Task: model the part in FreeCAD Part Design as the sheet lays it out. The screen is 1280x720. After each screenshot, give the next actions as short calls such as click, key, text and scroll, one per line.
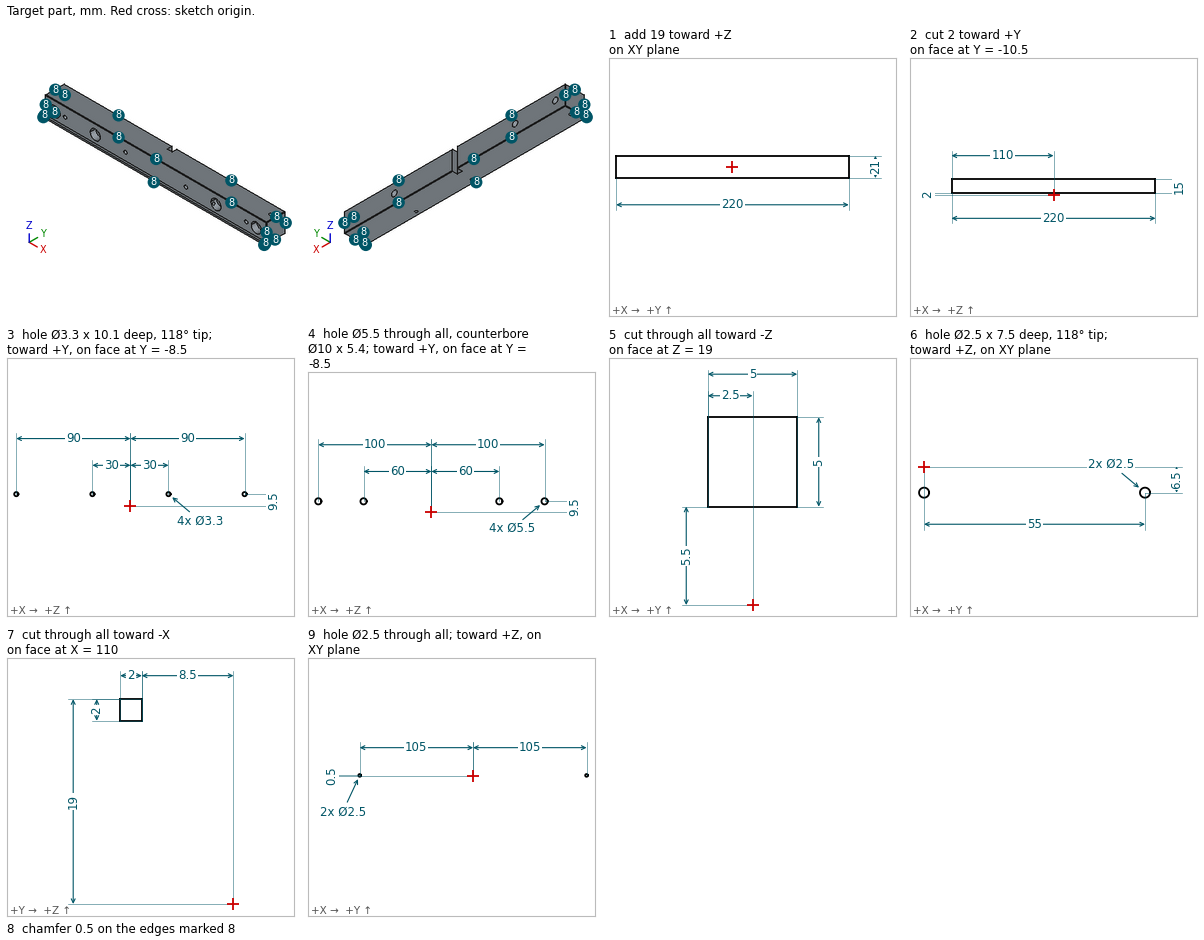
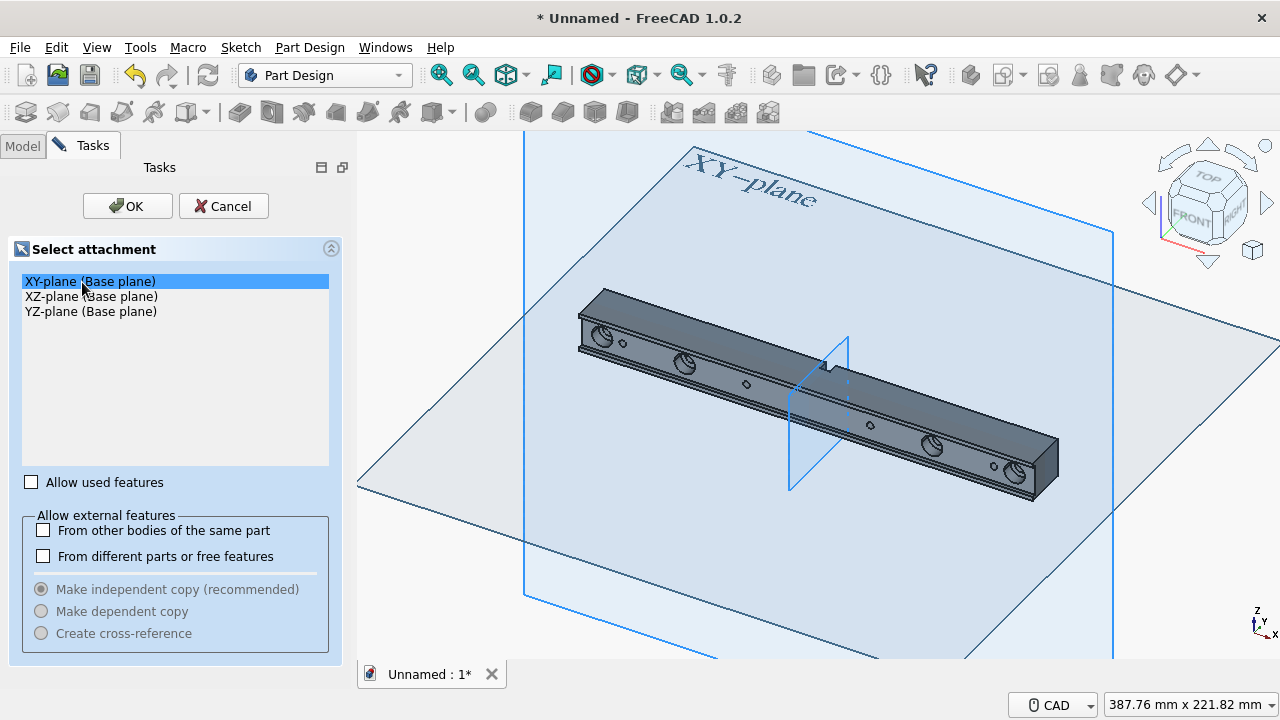
click(128, 206)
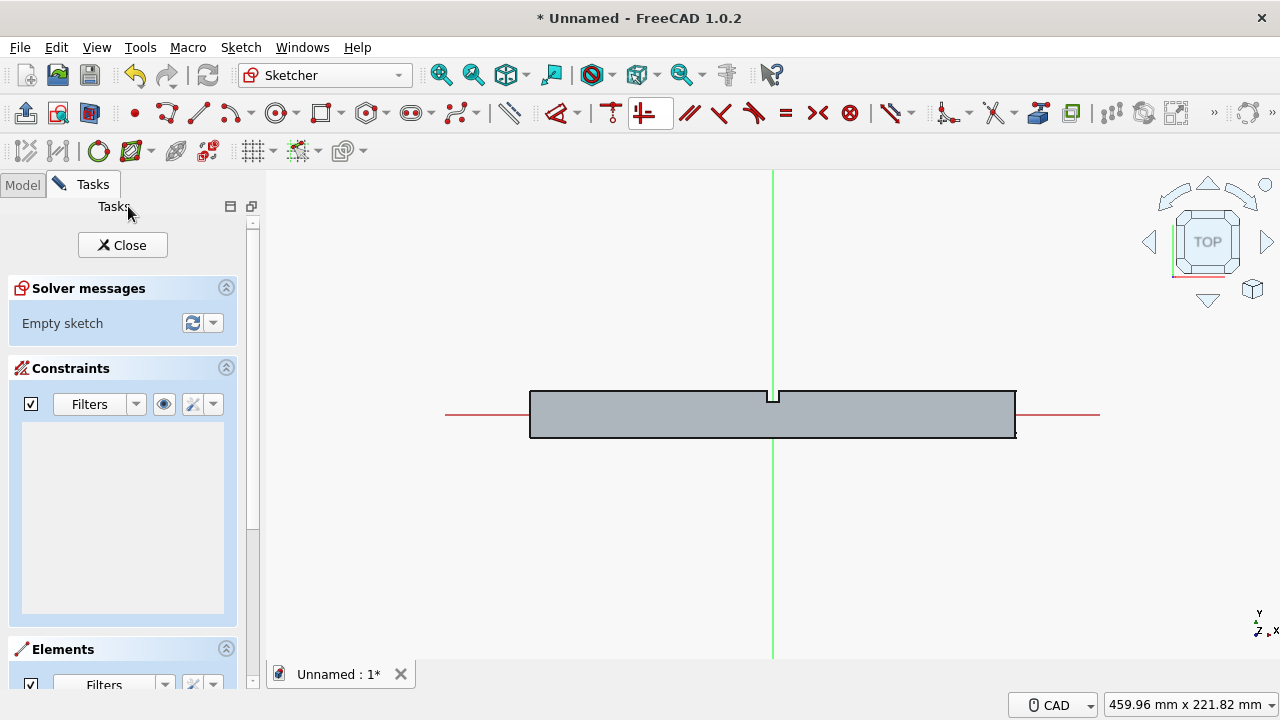
click(90, 114)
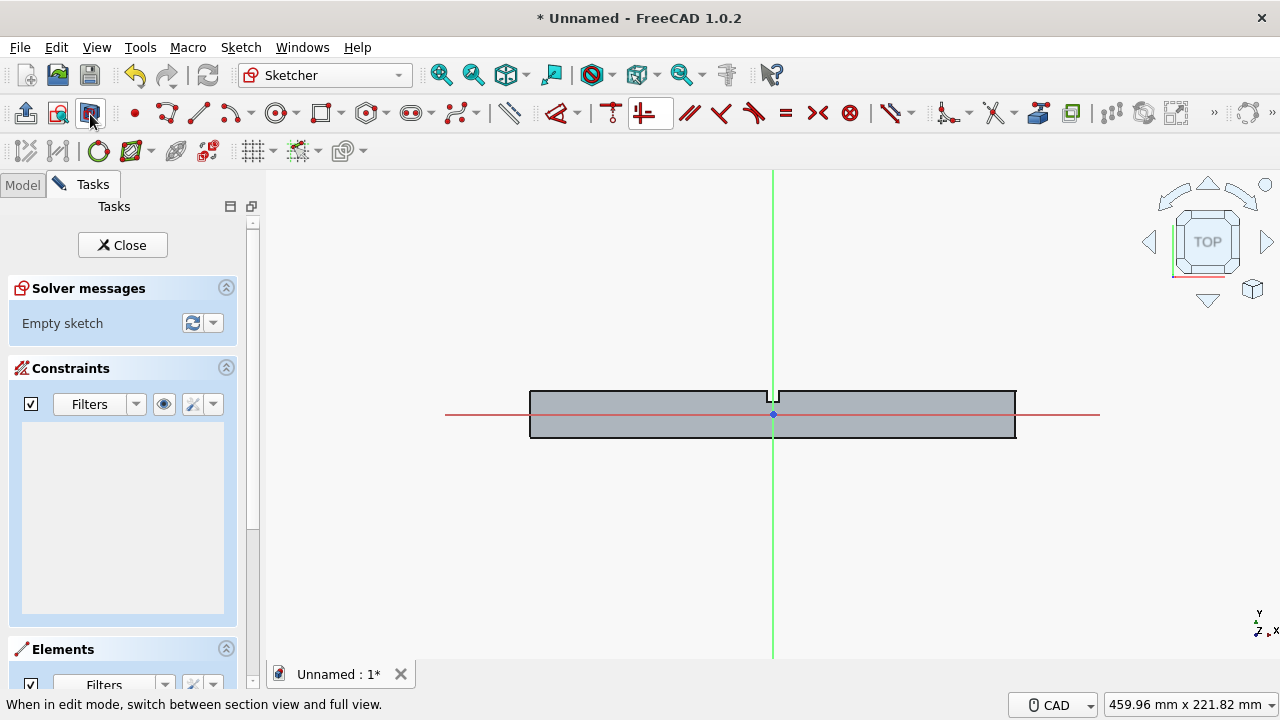
scroll(866, 425, up, 8)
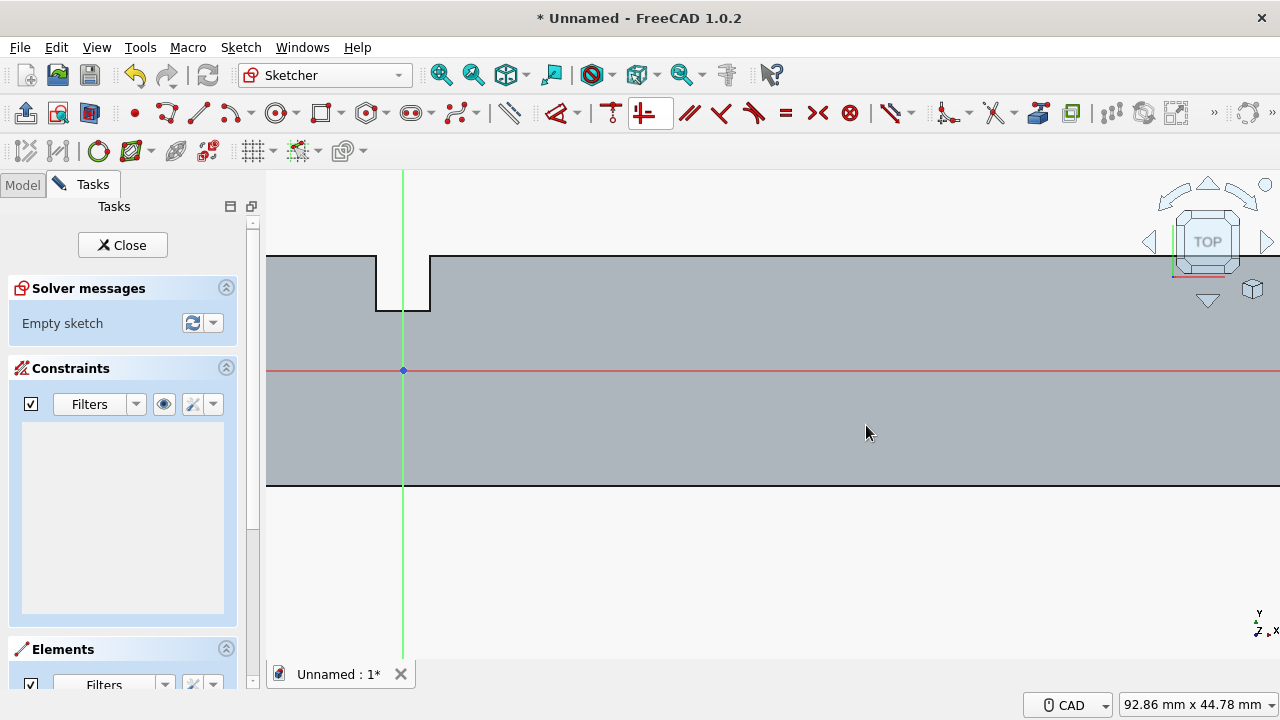
click(276, 114)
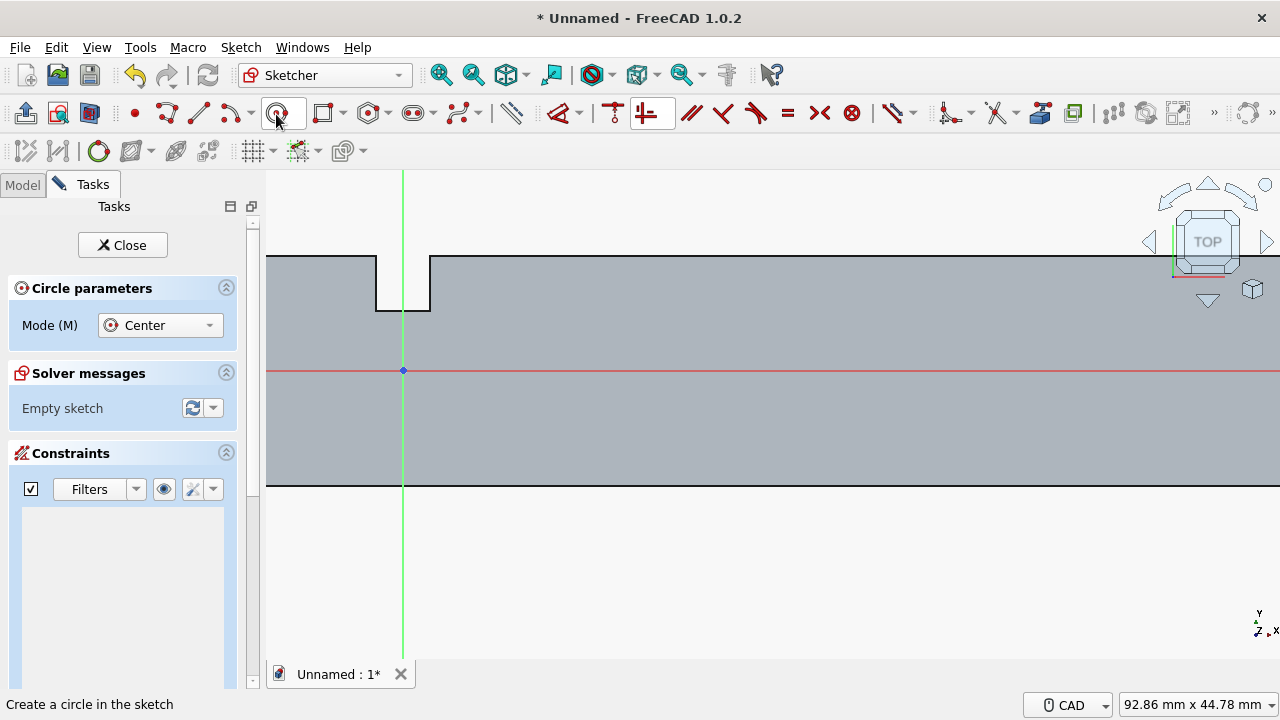
scroll(1004, 442, up, 3)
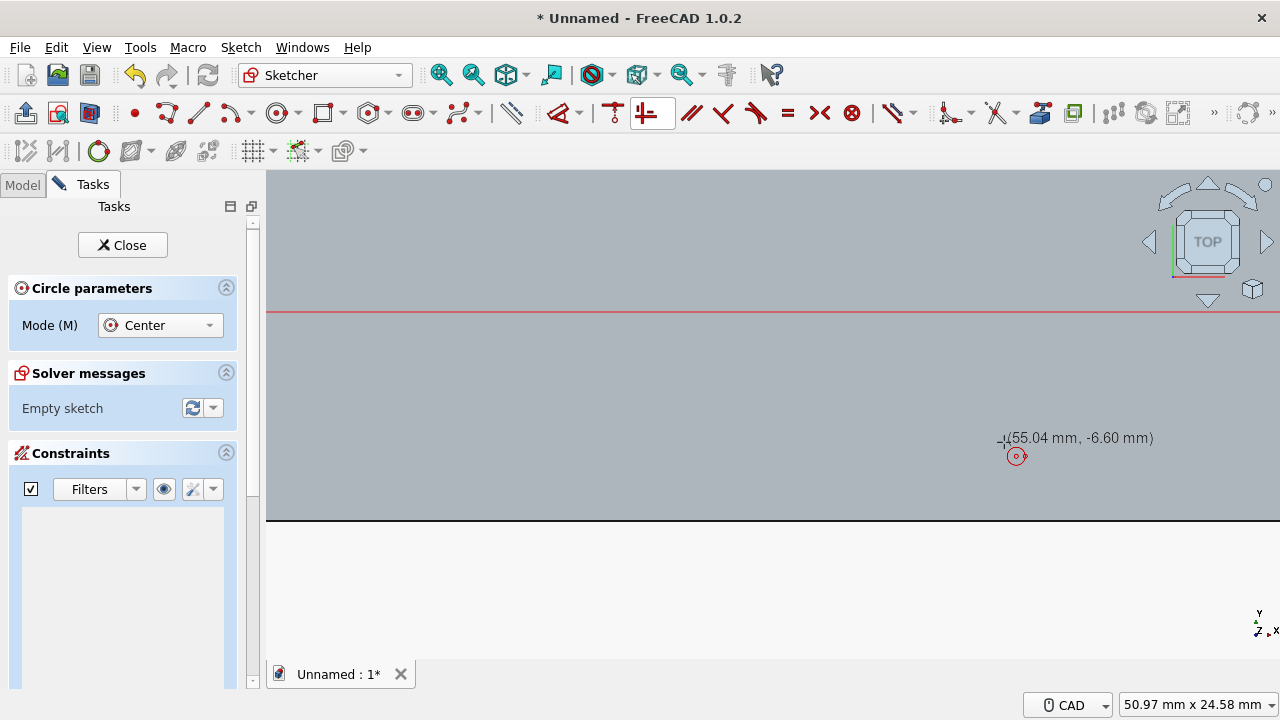
click(1003, 441)
move(1020, 424)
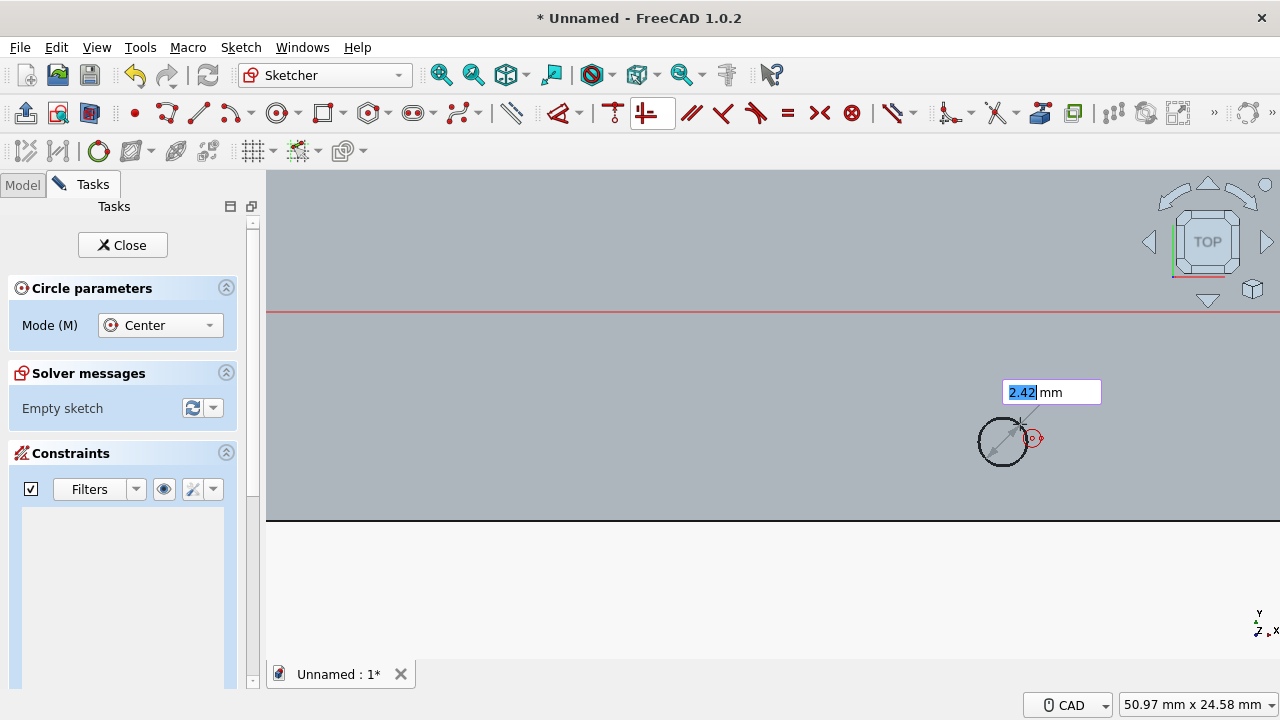
text(2.5)
key(Return)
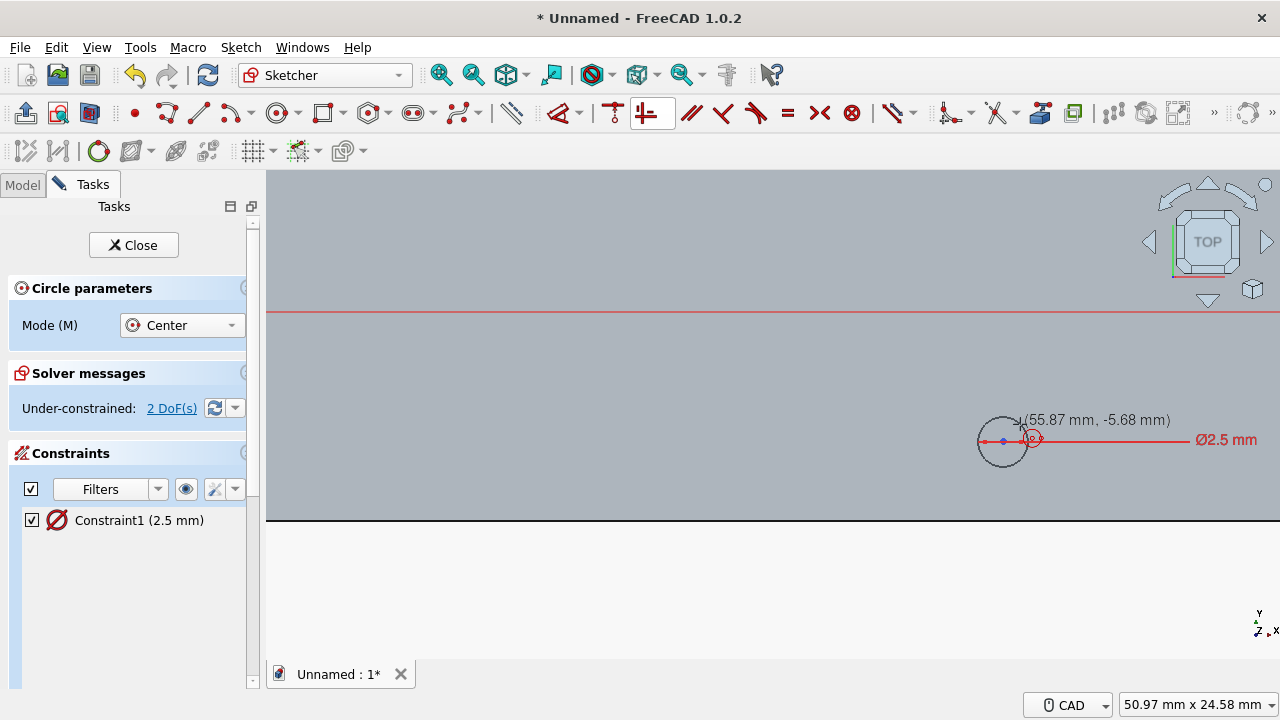
scroll(1007, 445, down, 3)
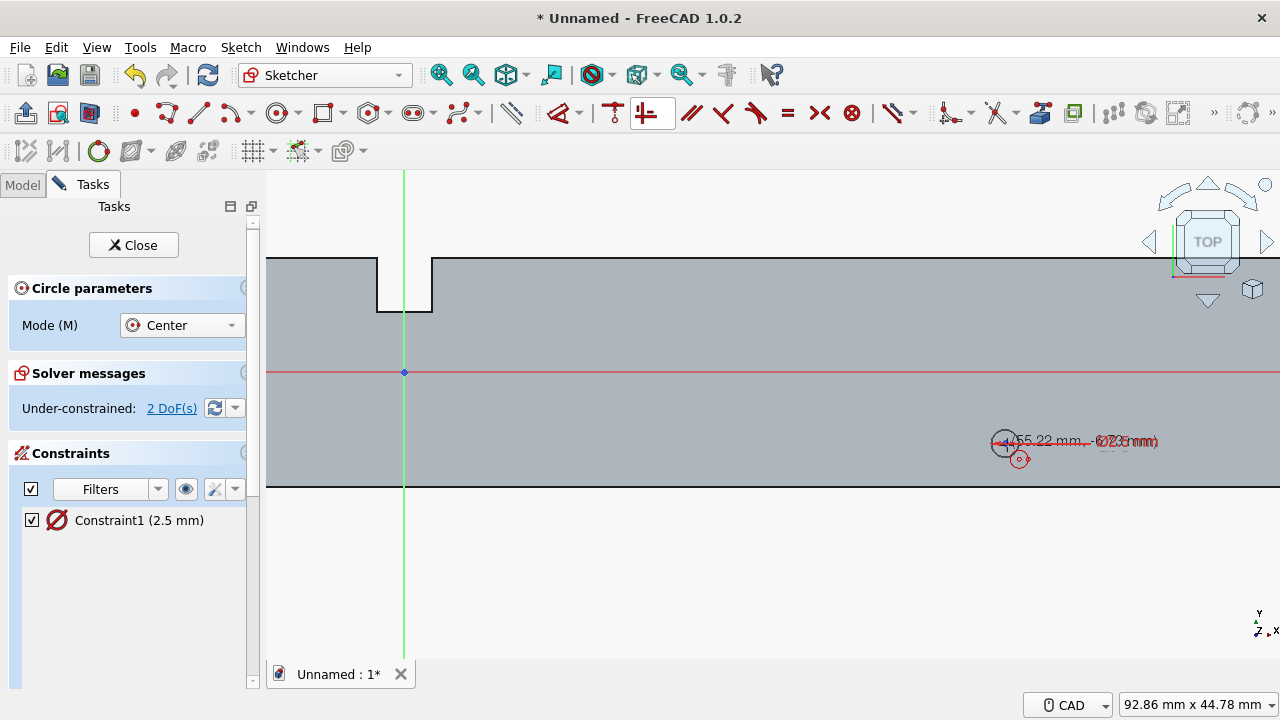
scroll(404, 443, up, 3)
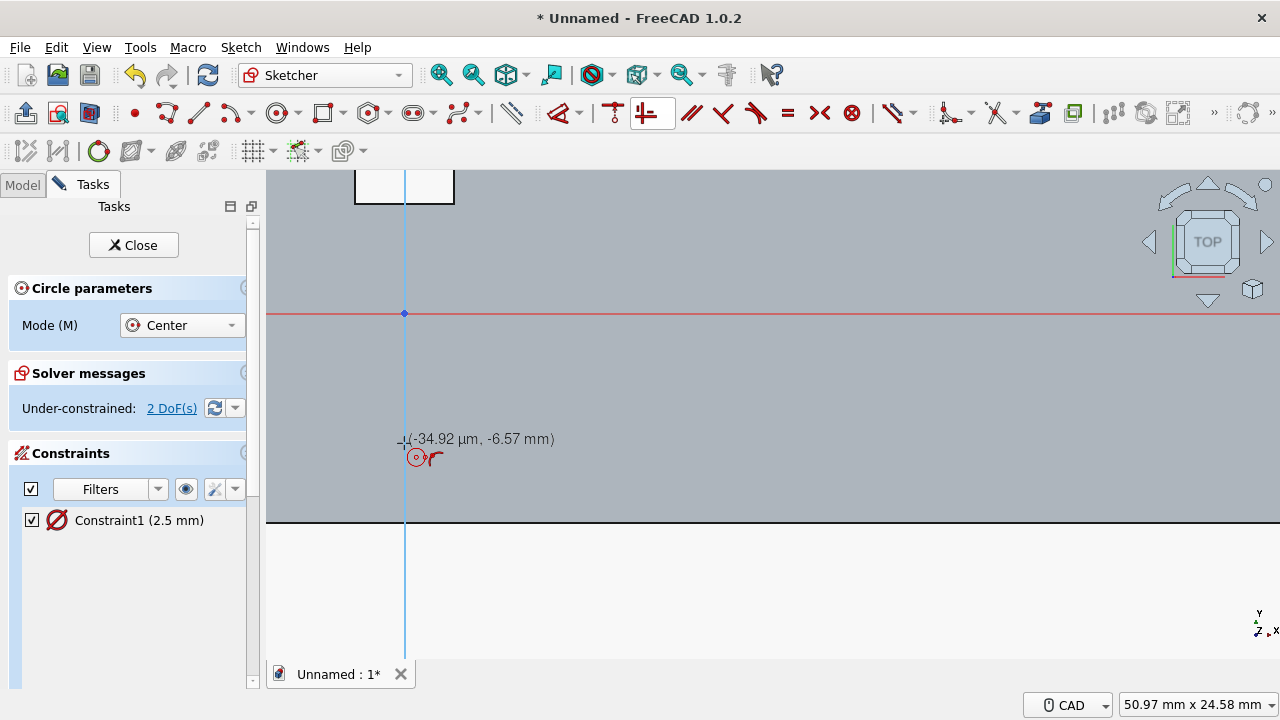
click(405, 443)
move(422, 425)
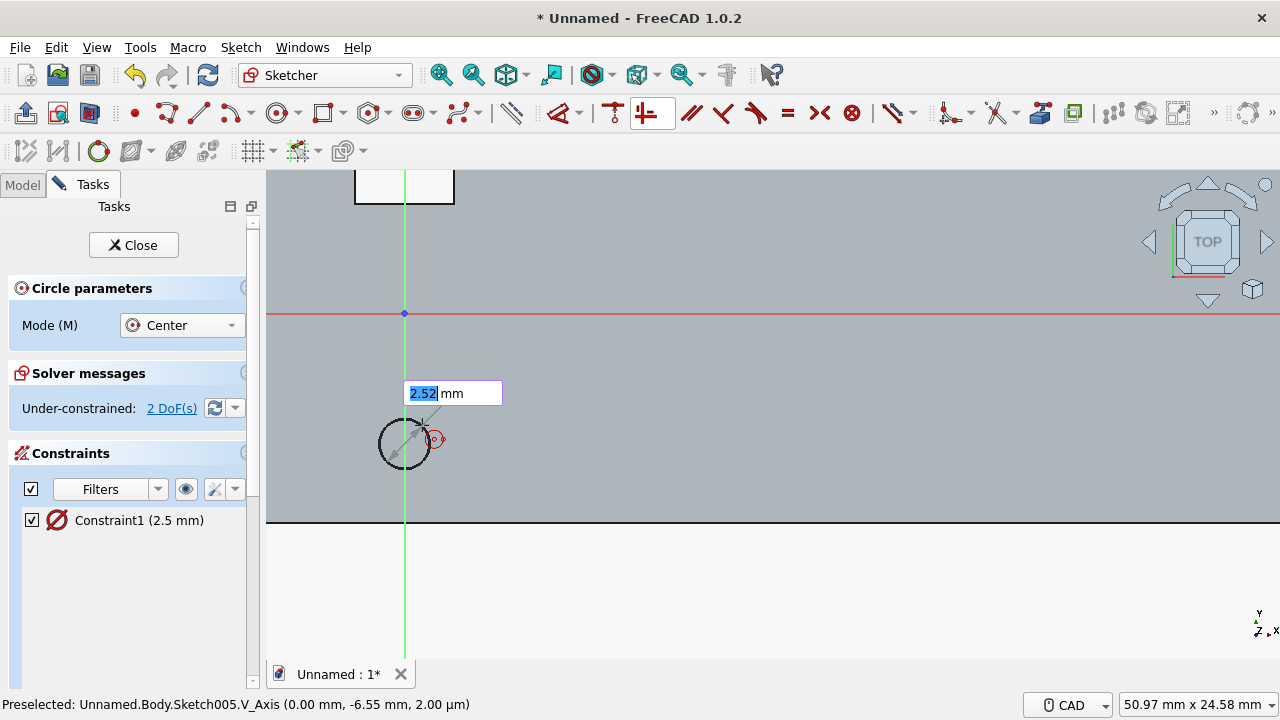
text(2.5)
key(Return)
key(Escape)